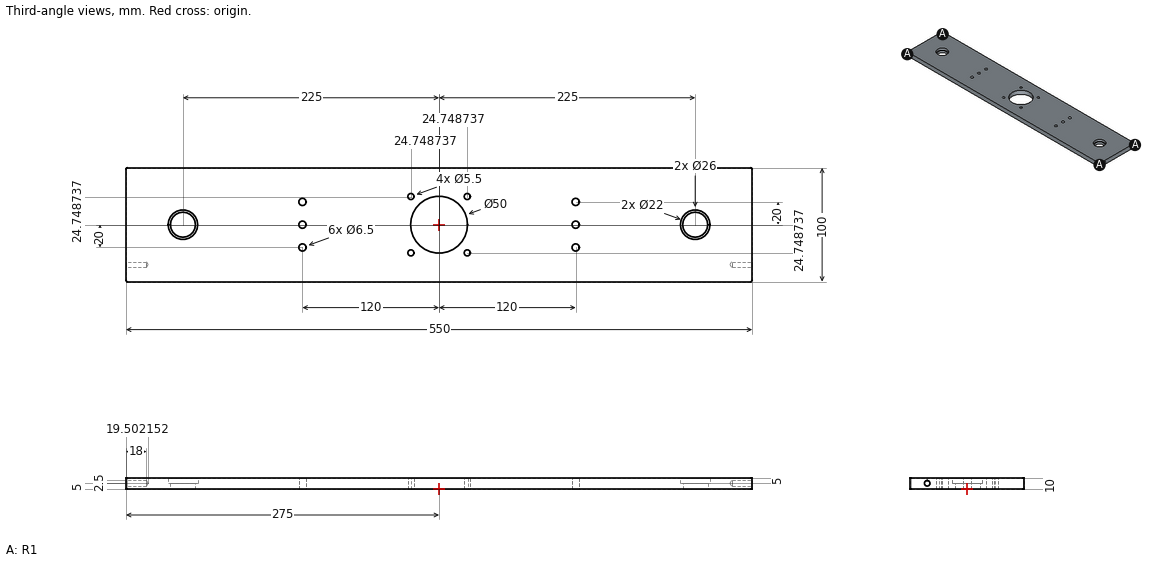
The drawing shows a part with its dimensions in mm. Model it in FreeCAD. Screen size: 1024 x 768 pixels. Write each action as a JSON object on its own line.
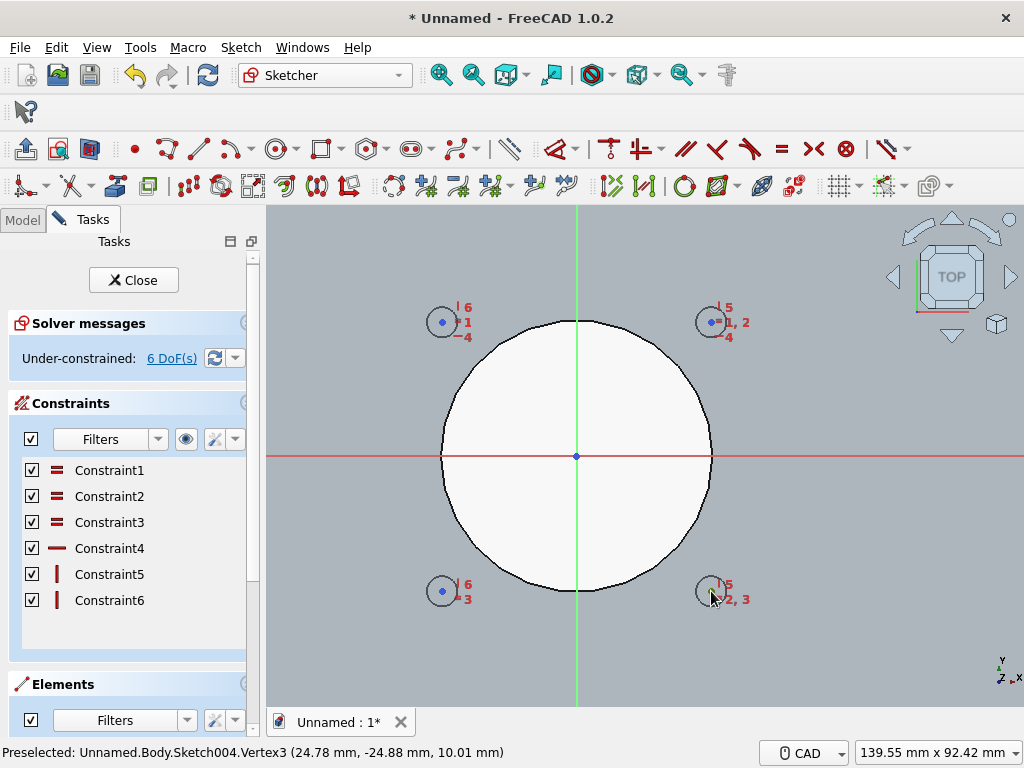
{"action": "left_click", "coordinate": [442, 591]}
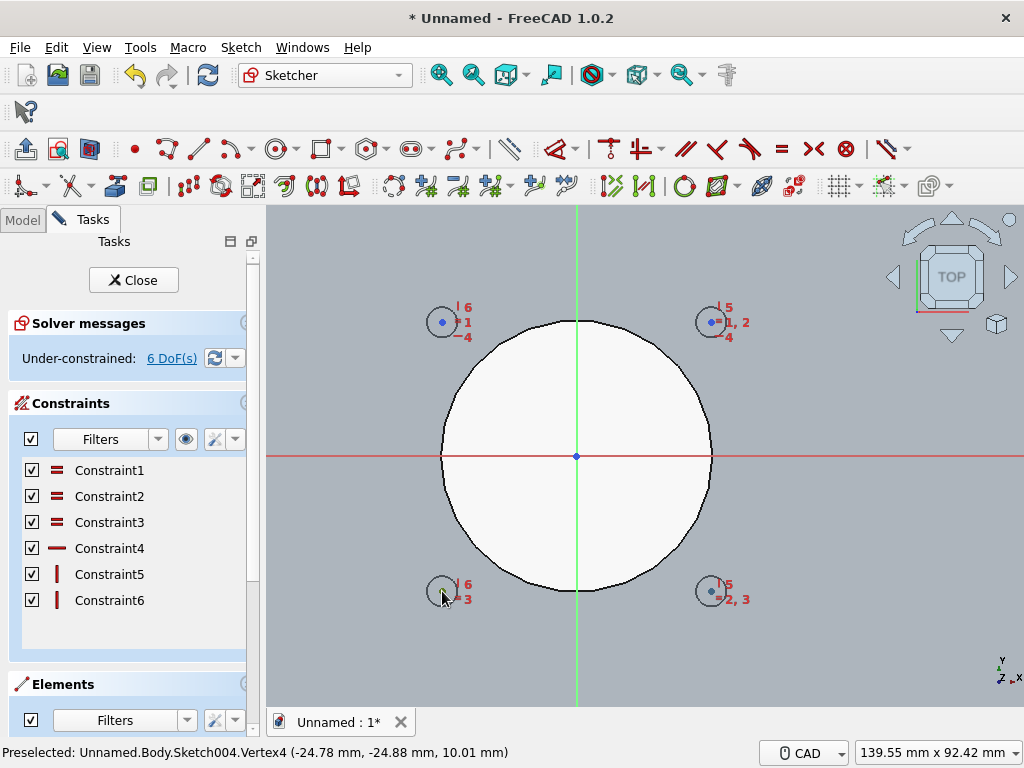
{"action": "key", "text": "h"}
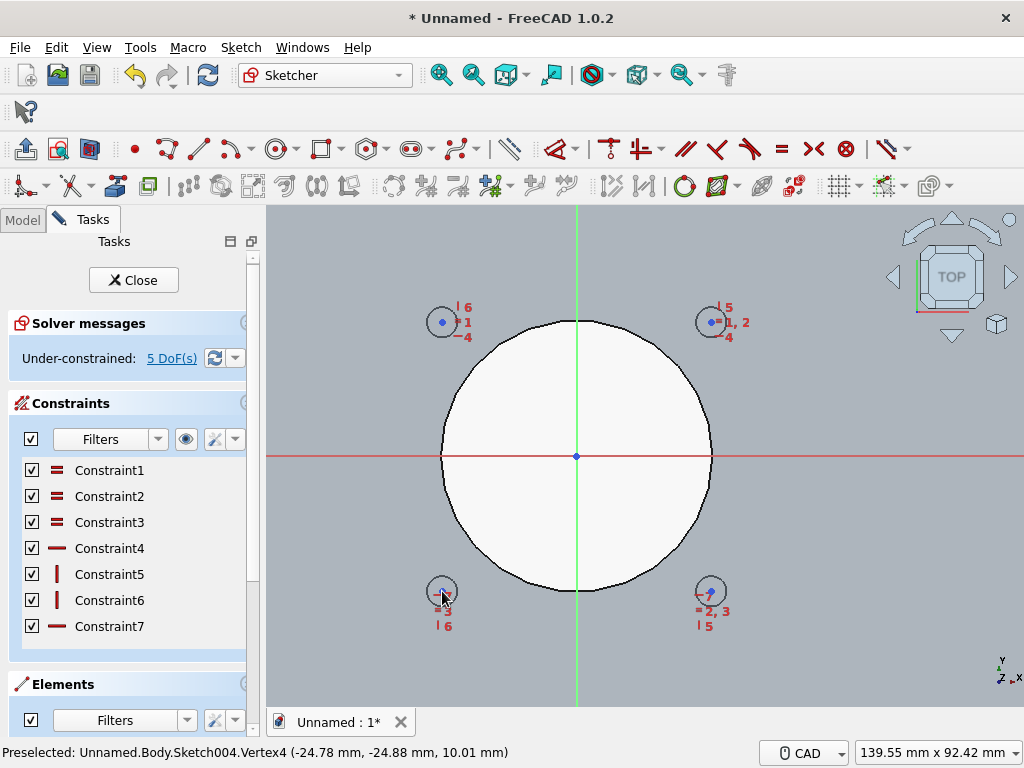
{"action": "key", "text": "d"}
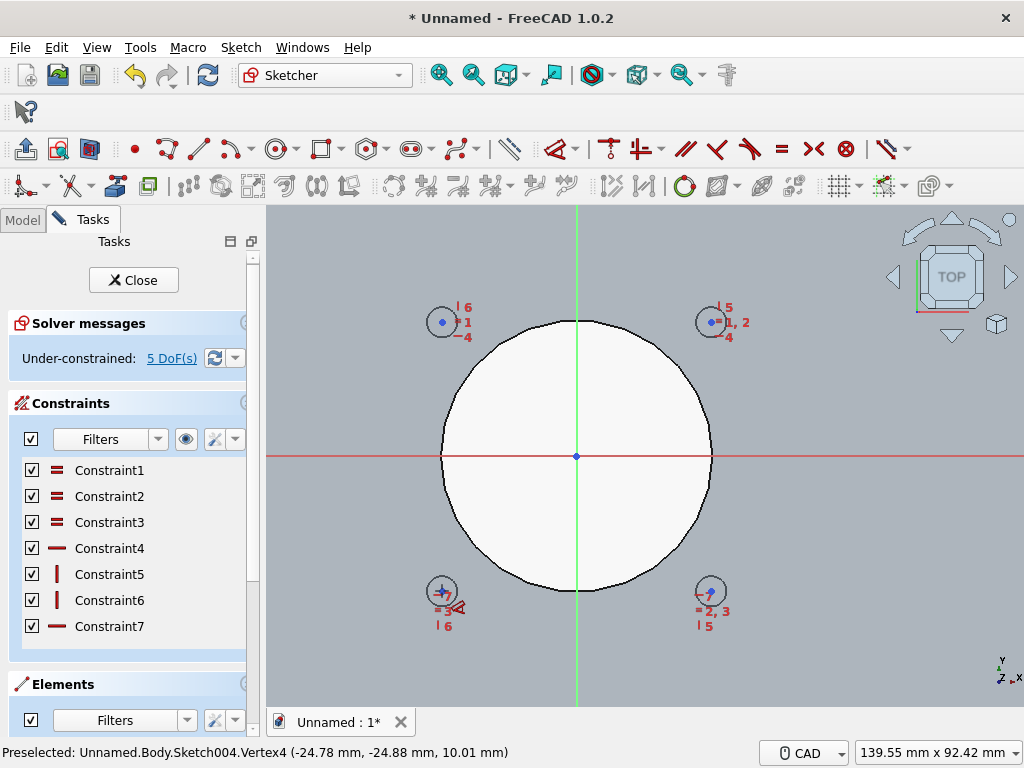
{"action": "scroll", "coordinate": [453, 312], "scroll_direction": "up", "scroll_amount": 2}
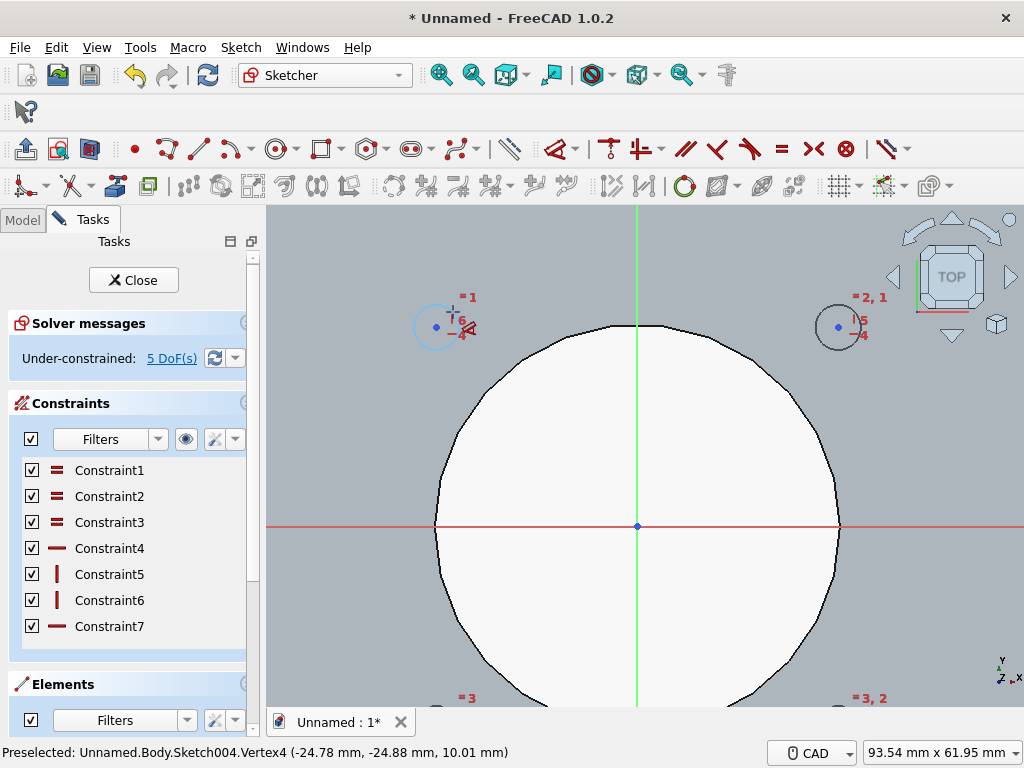
{"action": "left_click", "coordinate": [452, 311]}
{"action": "left_click", "coordinate": [474, 288]}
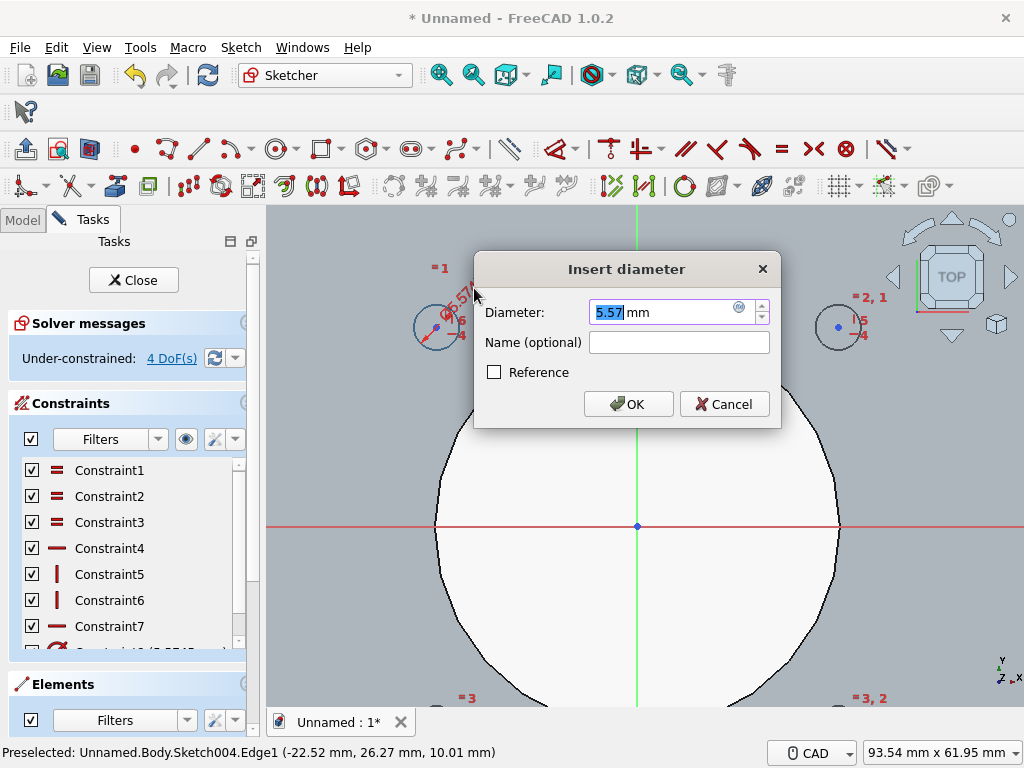
{"action": "type", "text": "5.5"}
{"action": "key", "text": "Return"}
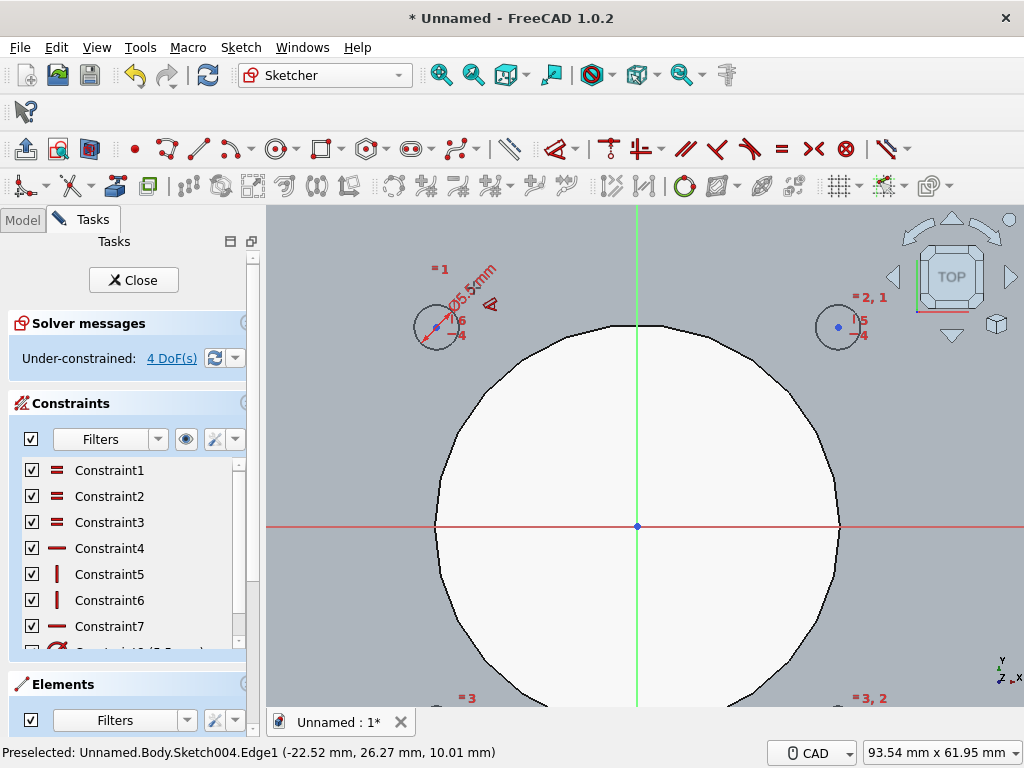
{"action": "left_click", "coordinate": [437, 327]}
{"action": "left_click", "coordinate": [583, 293]}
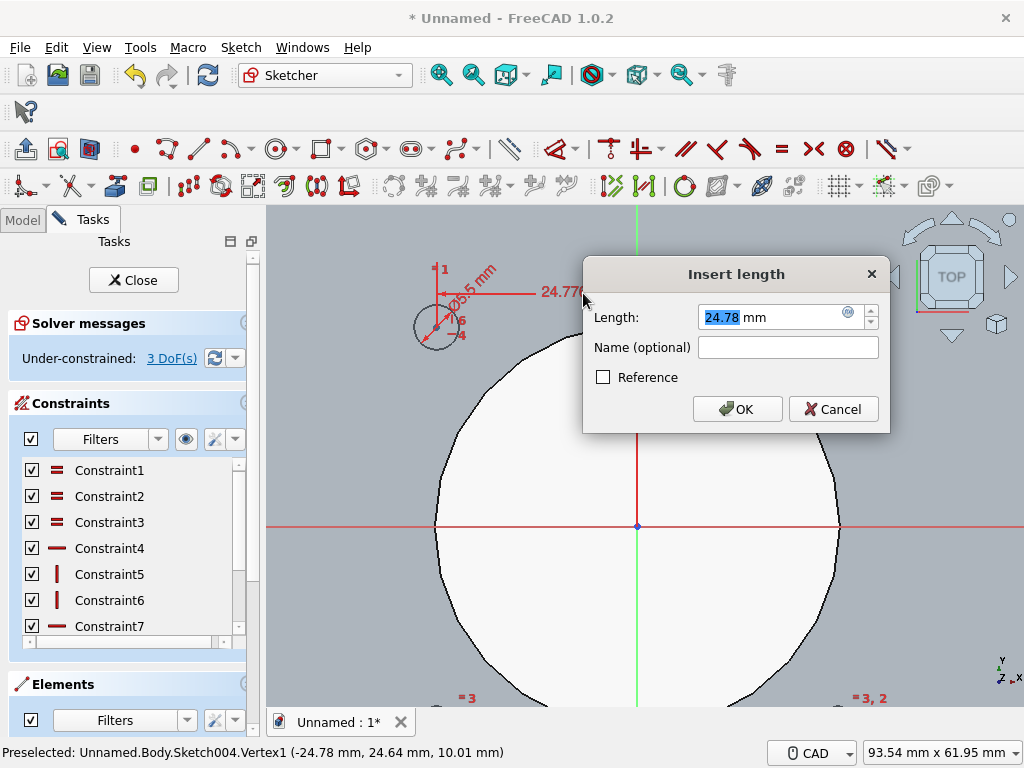
{"action": "type", "text": "24.748737"}
{"action": "key", "text": "Return"}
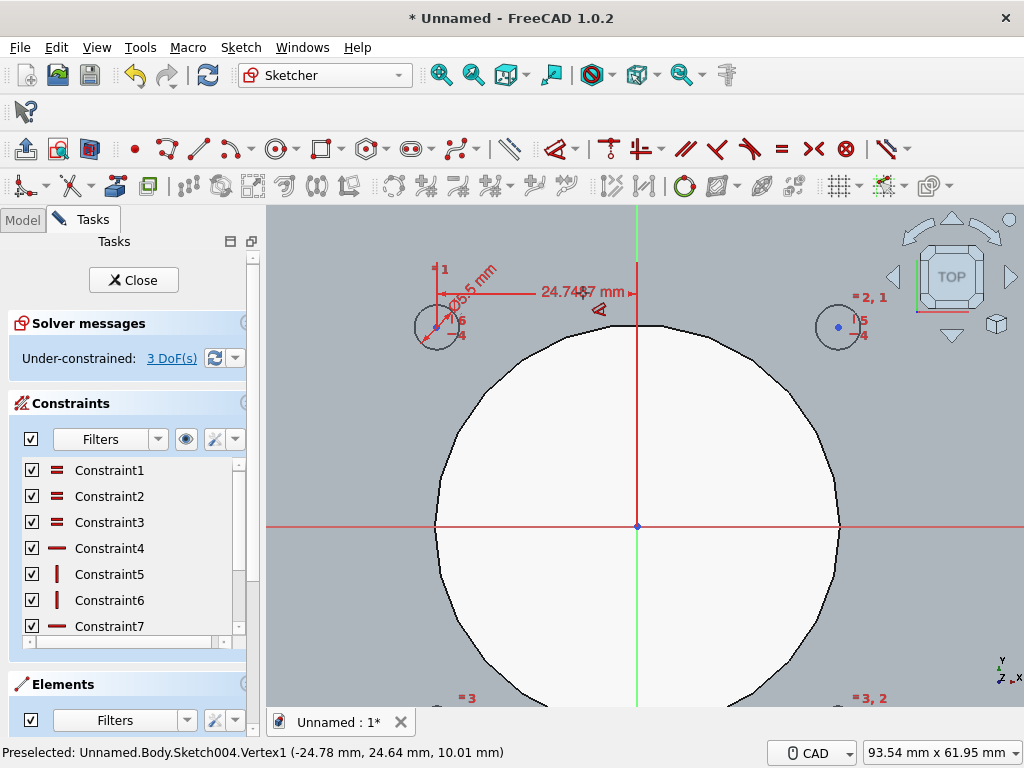
{"action": "left_click", "coordinate": [437, 327]}
{"action": "left_click", "coordinate": [403, 427]}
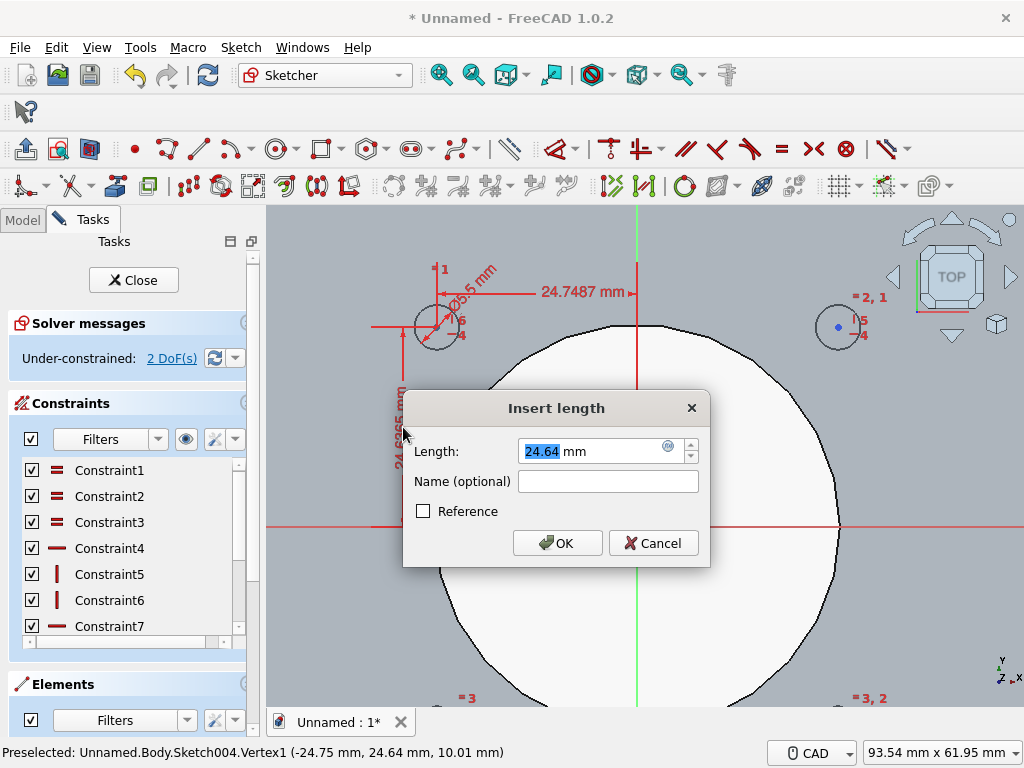
{"action": "type", "text": "24.748737"}
{"action": "key", "text": "Return"}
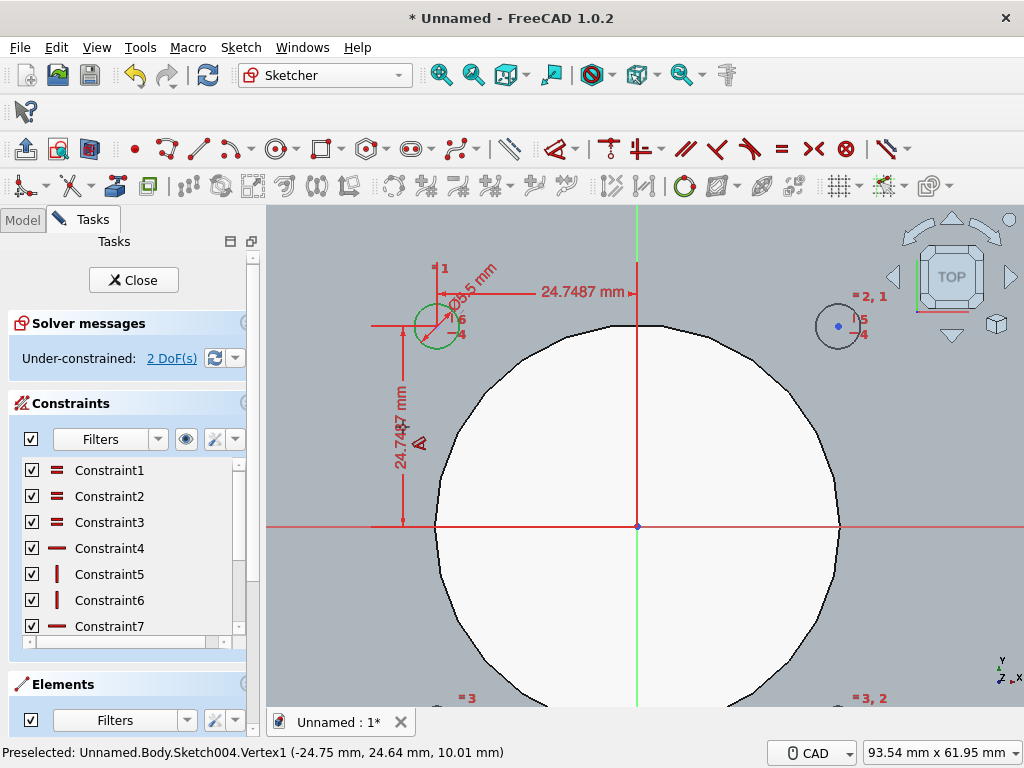
{"action": "left_click", "coordinate": [838, 326]}
{"action": "left_click", "coordinate": [738, 292]}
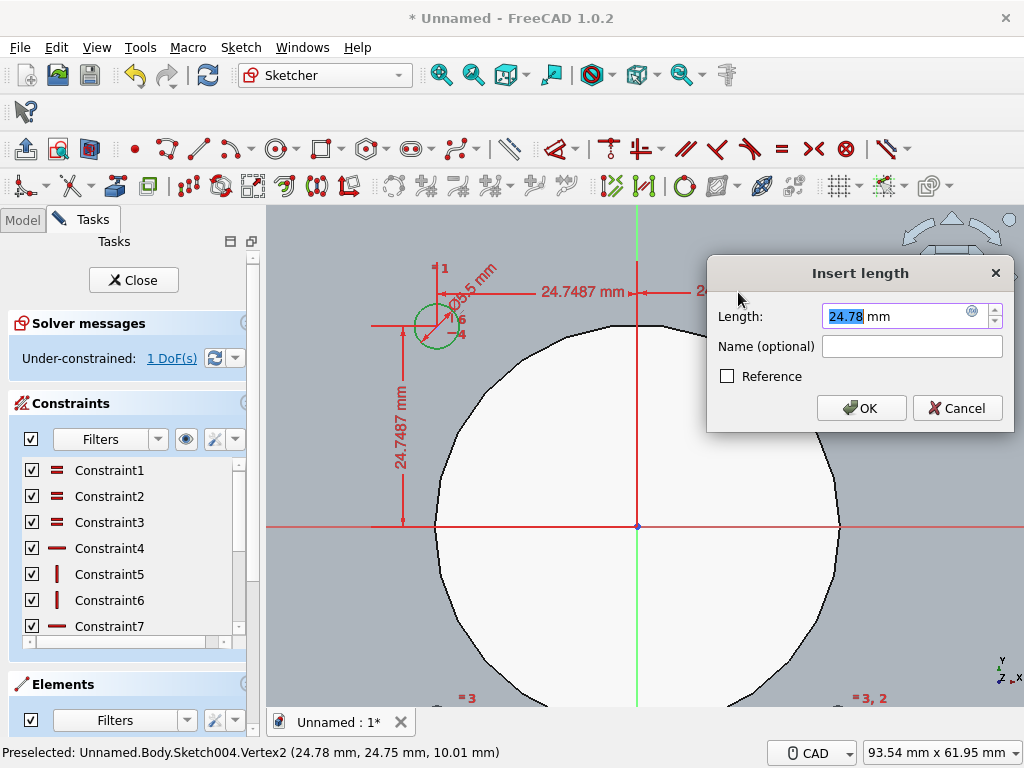
{"action": "type", "text": "24.748737"}
{"action": "key", "text": "Return"}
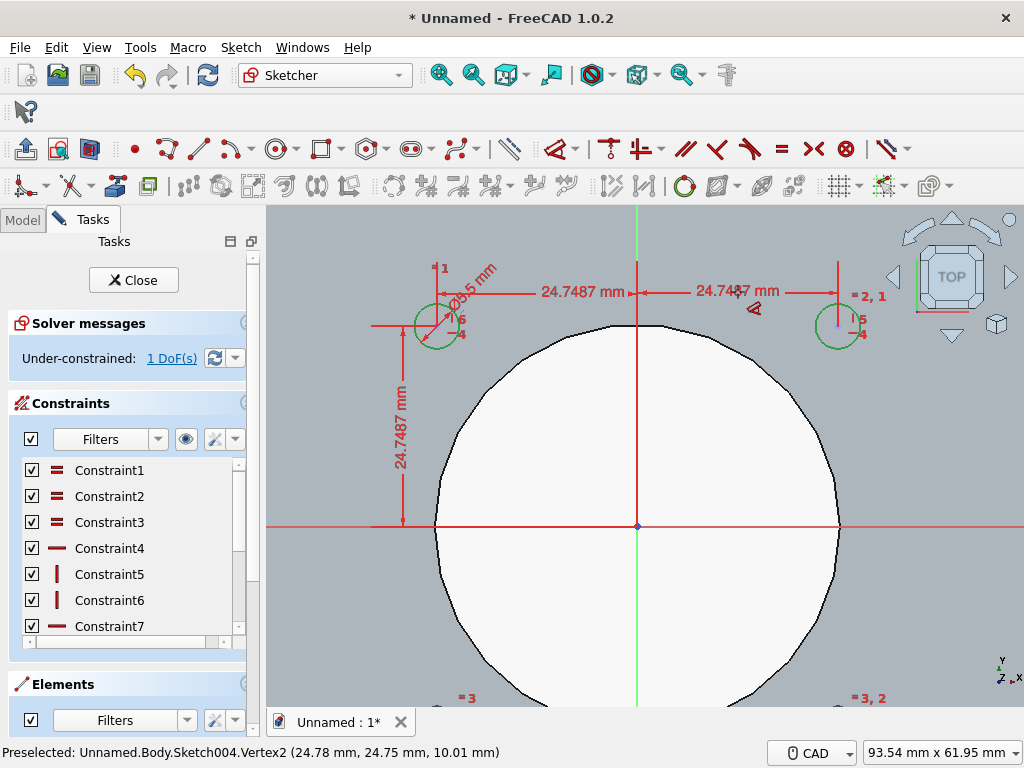
{"action": "scroll", "coordinate": [453, 312], "scroll_direction": "down", "scroll_amount": 2}